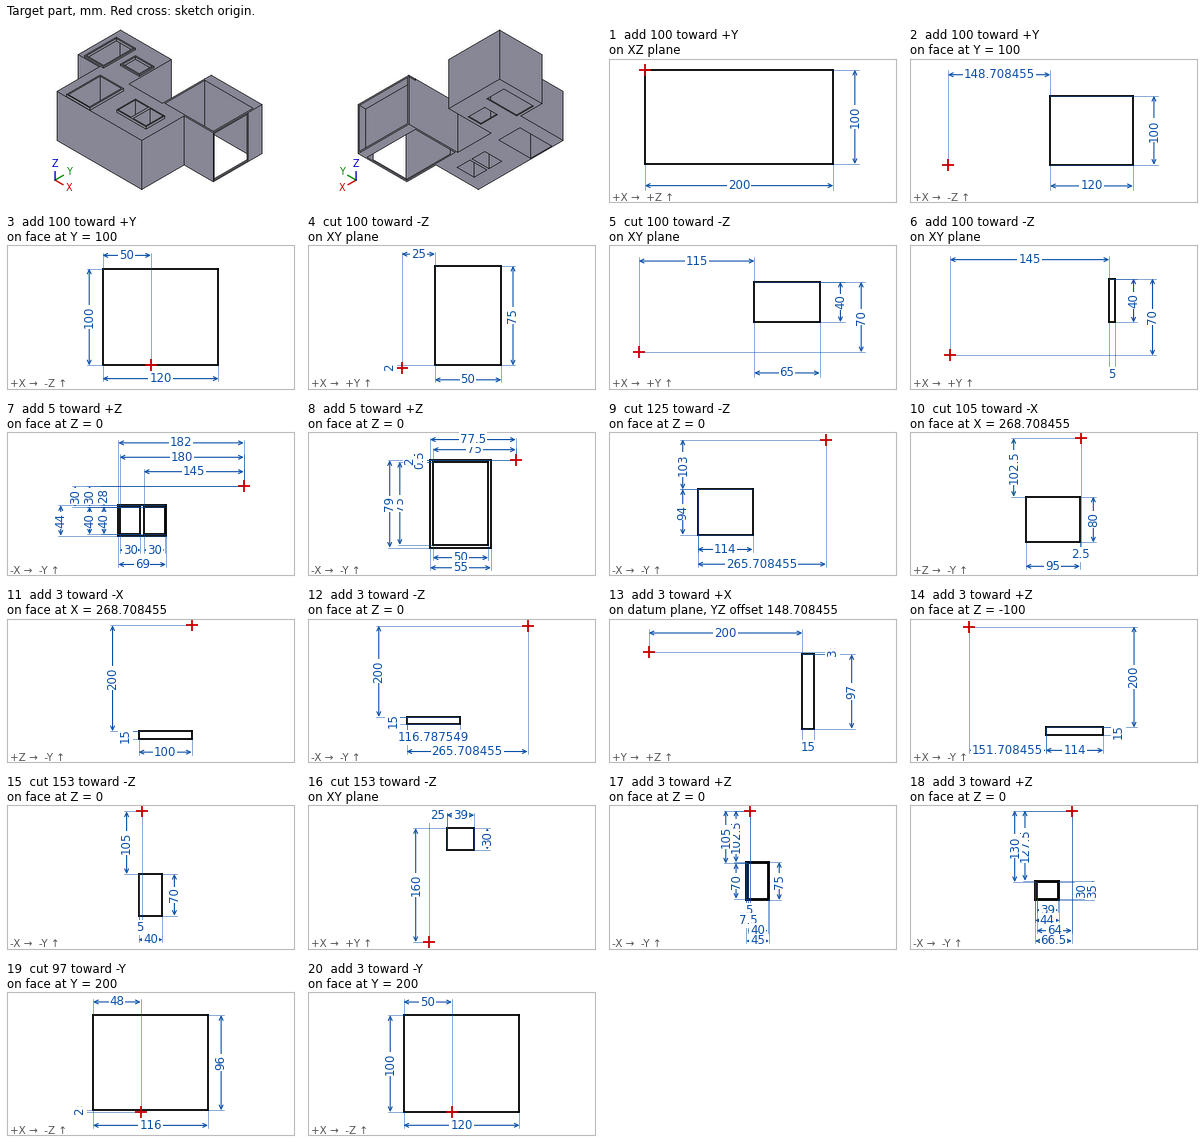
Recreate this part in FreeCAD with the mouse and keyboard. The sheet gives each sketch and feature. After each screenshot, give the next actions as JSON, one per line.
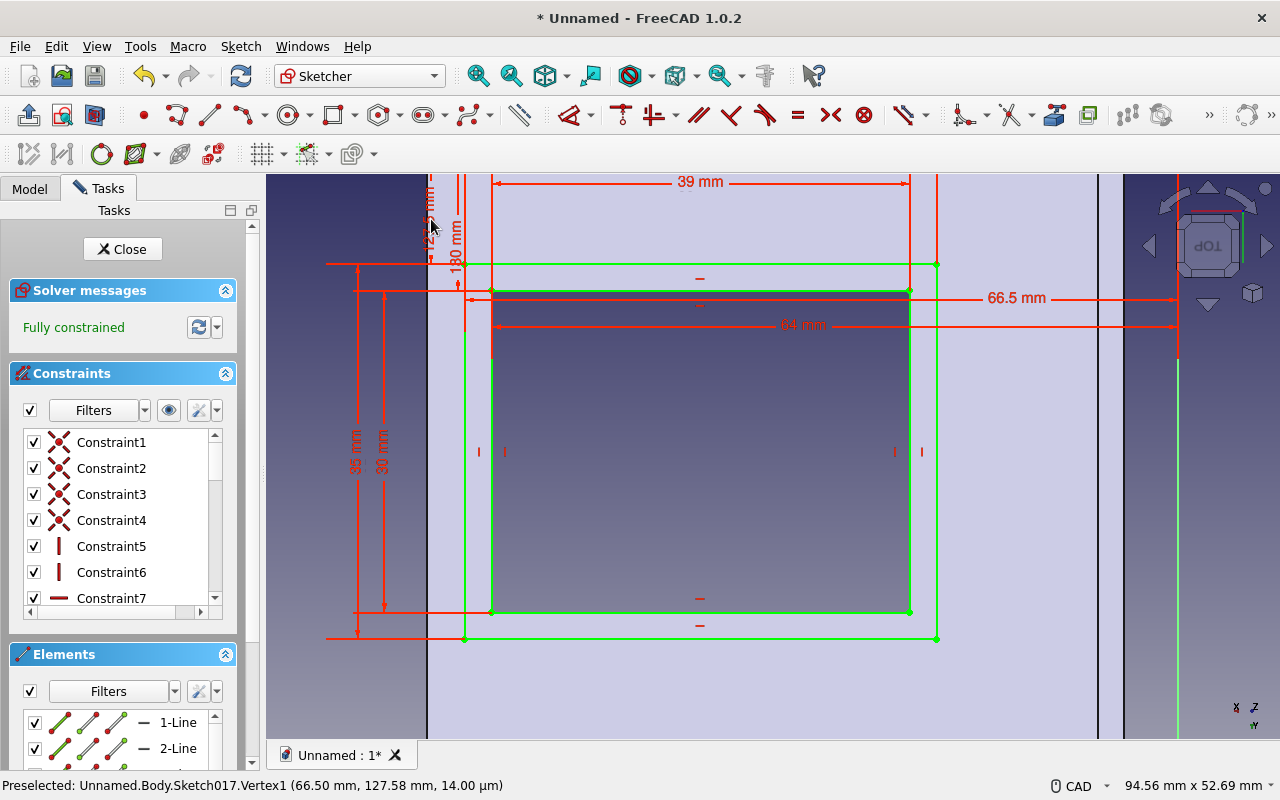
{"action": "left_click", "coordinate": [123, 249]}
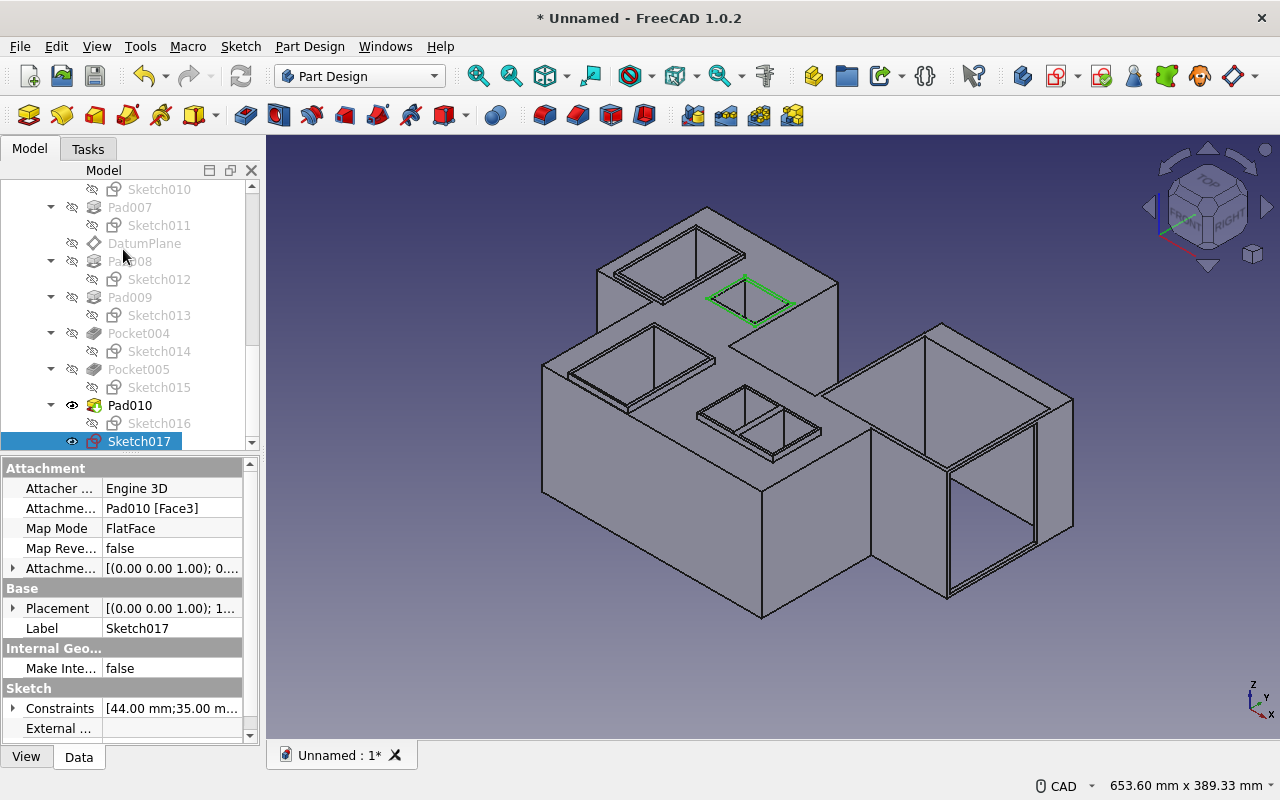
{"action": "left_click", "coordinate": [29, 116]}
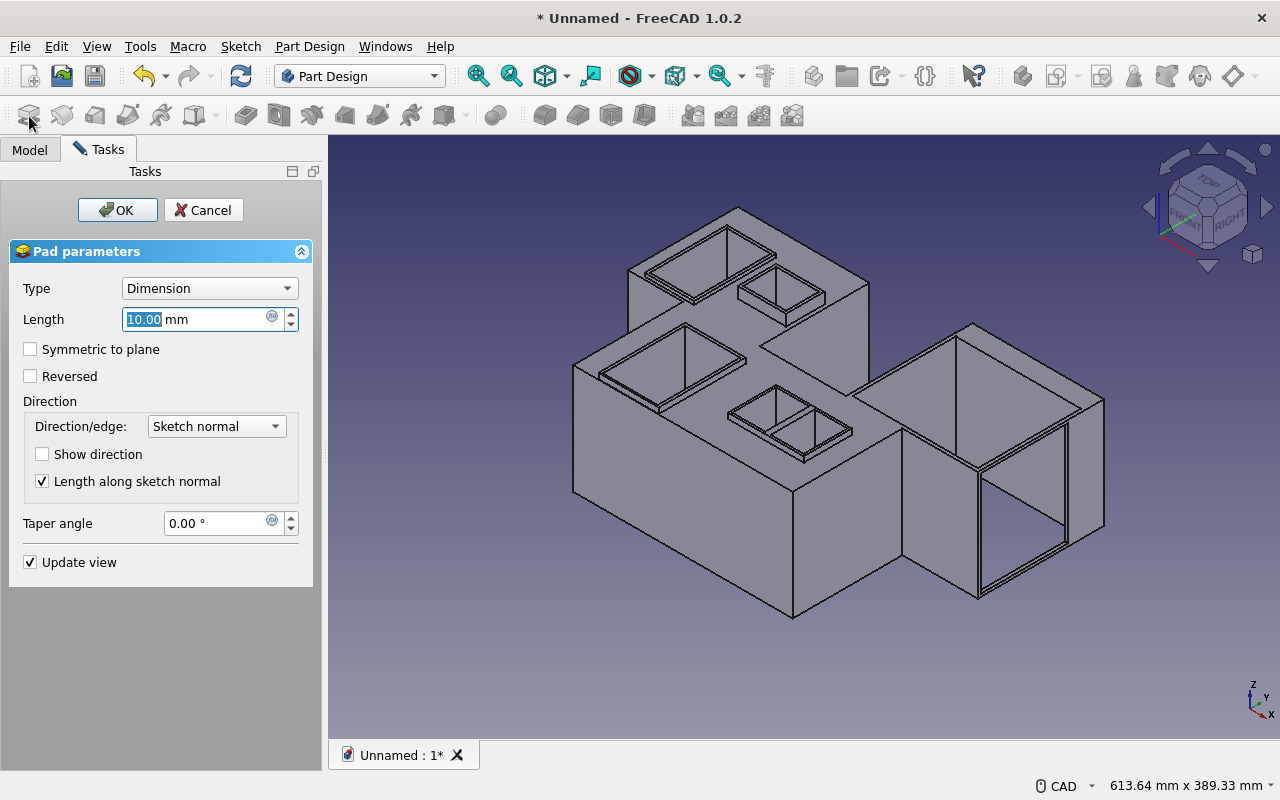
{"action": "type", "text": "3"}
{"action": "key", "text": "Tab"}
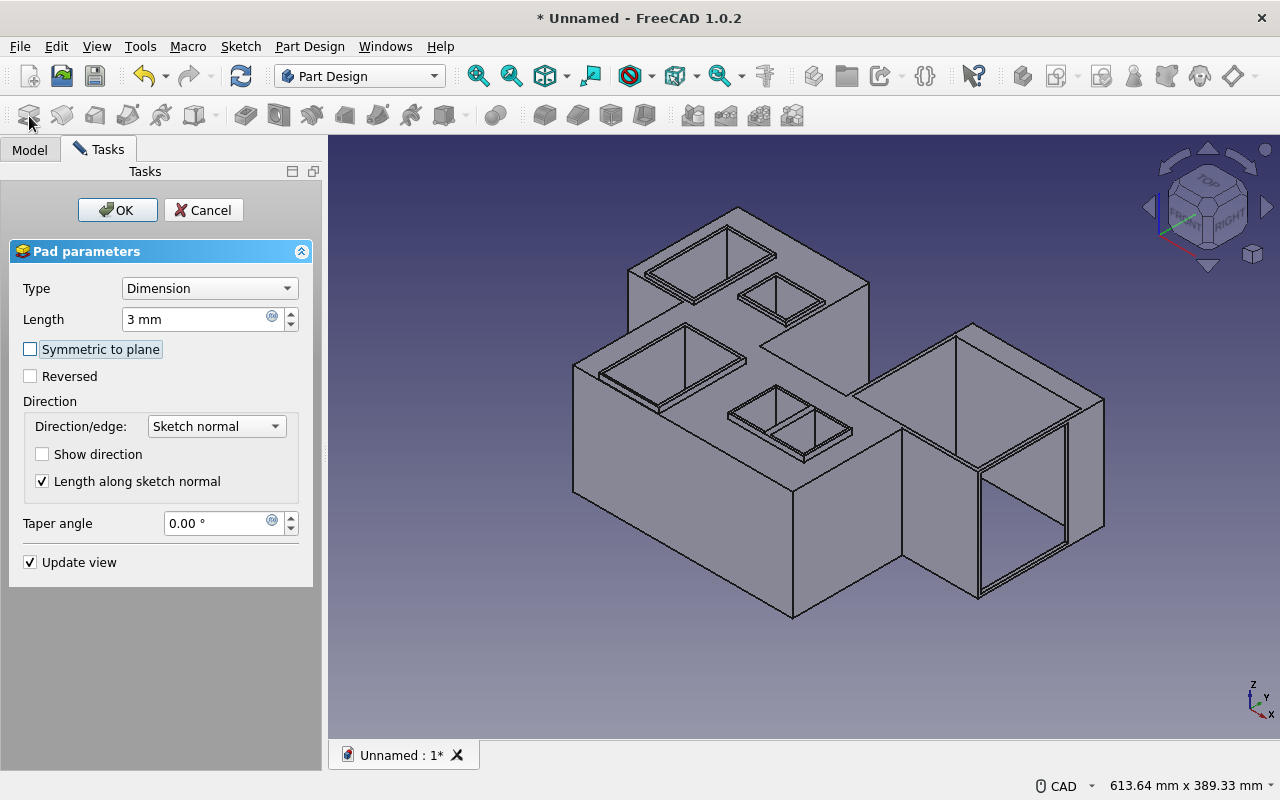
{"action": "left_click", "coordinate": [118, 210]}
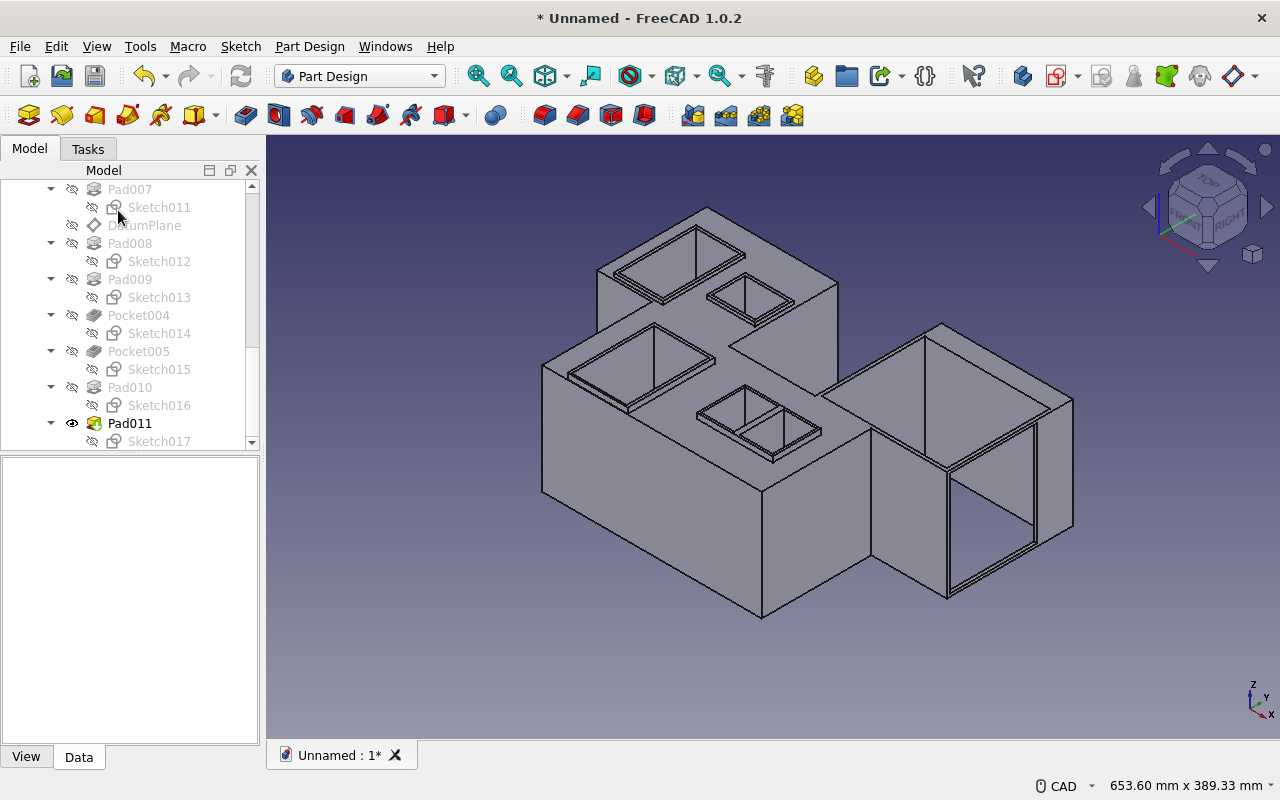
{"action": "key", "text": "4"}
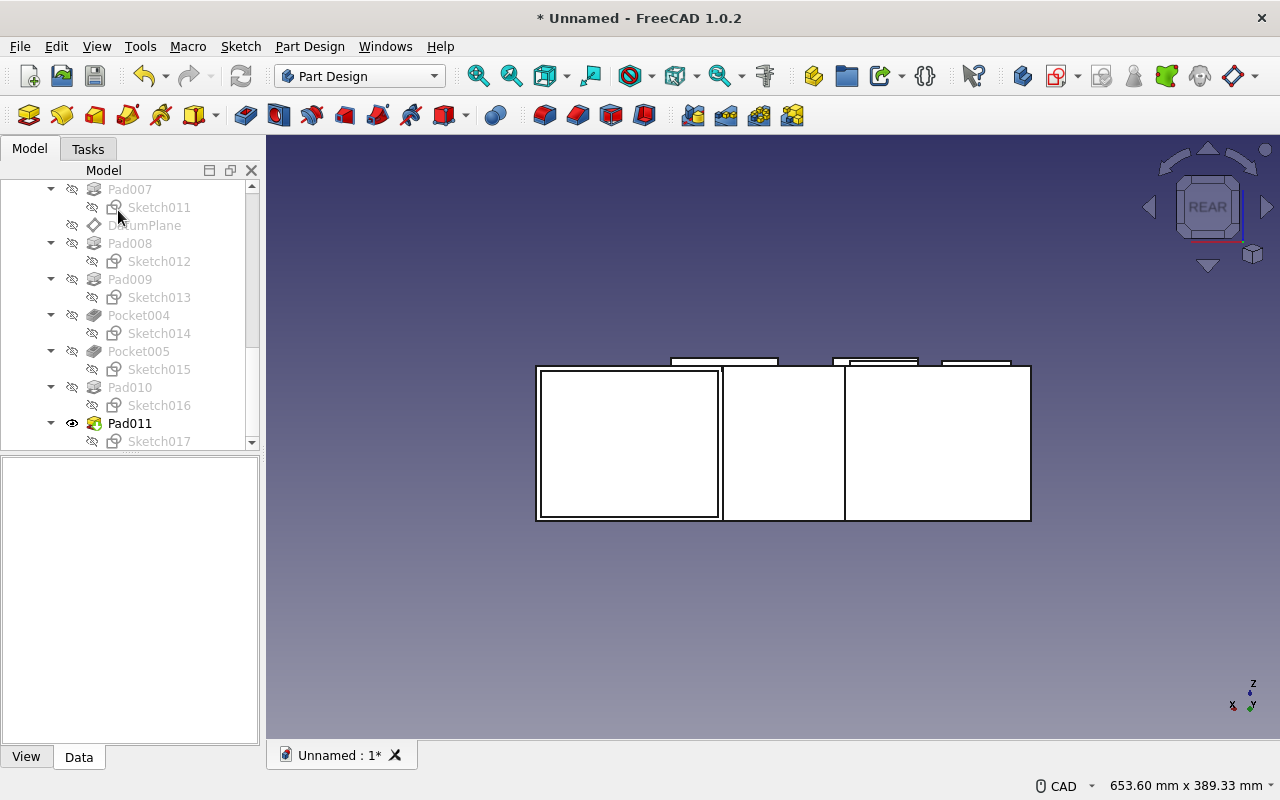
{"action": "left_click", "coordinate": [938, 443]}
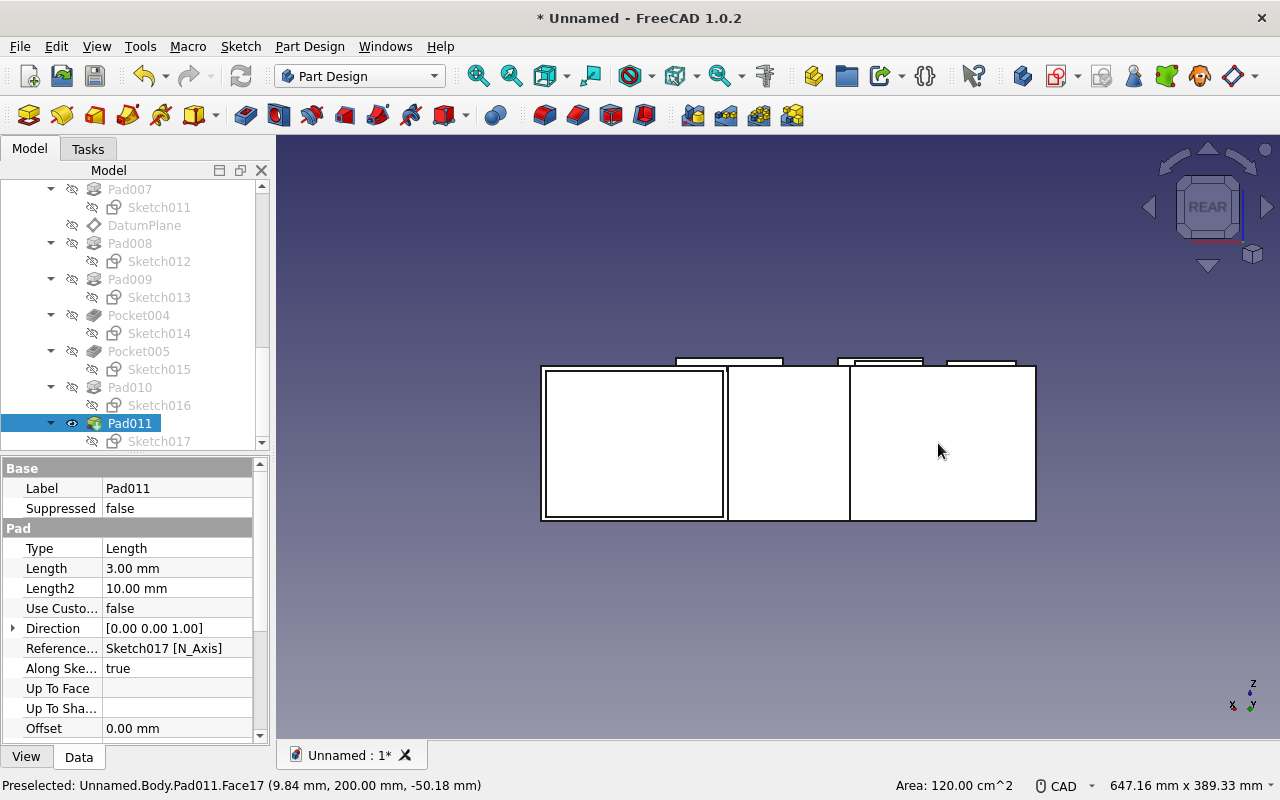
{"action": "left_click", "coordinate": [1056, 76]}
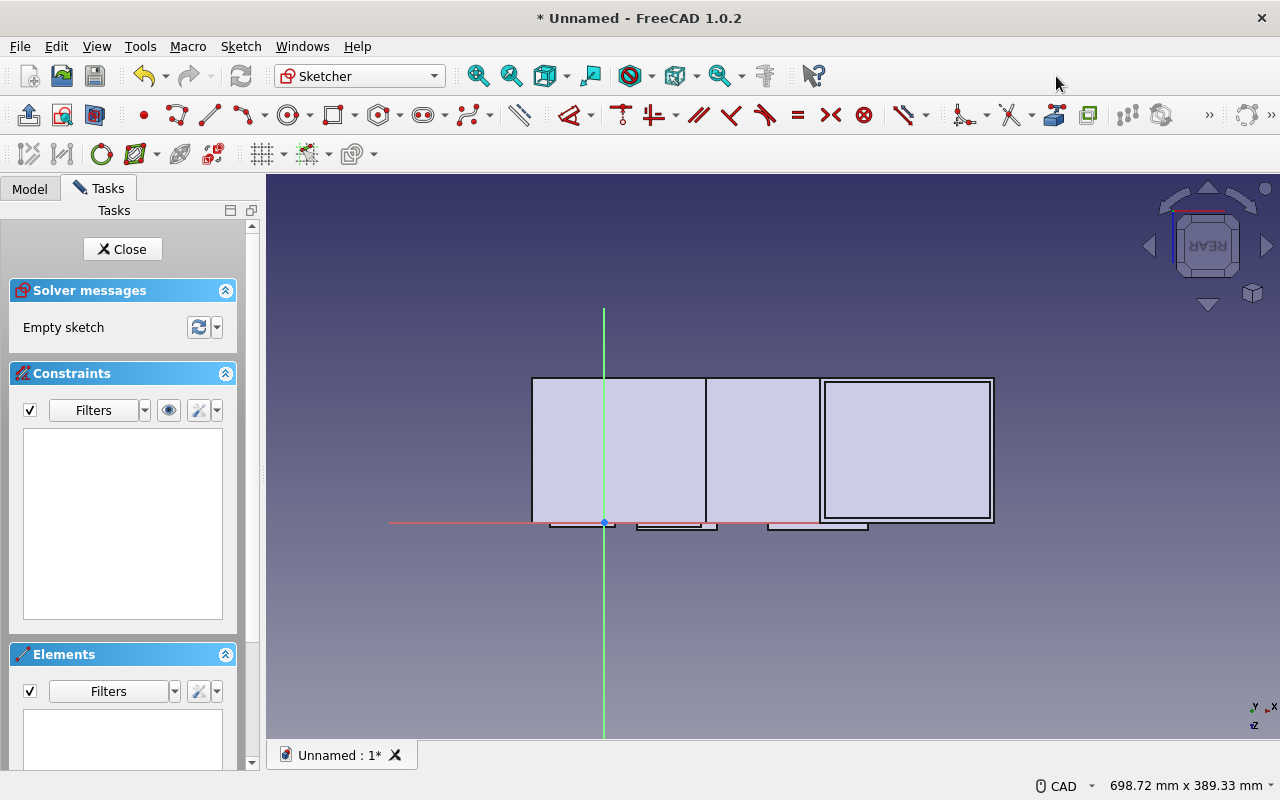
{"action": "left_click", "coordinate": [95, 116]}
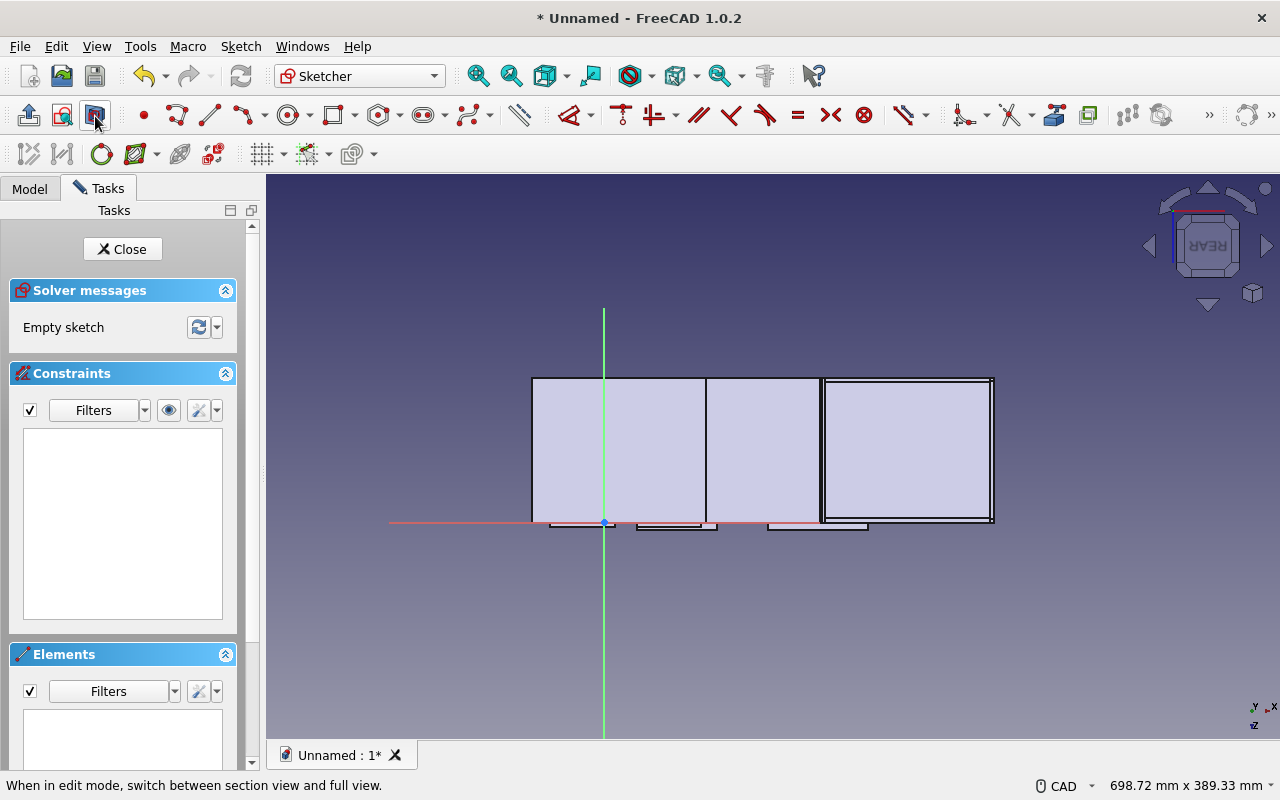
{"action": "scroll", "coordinate": [569, 449], "scroll_direction": "up", "scroll_amount": 5}